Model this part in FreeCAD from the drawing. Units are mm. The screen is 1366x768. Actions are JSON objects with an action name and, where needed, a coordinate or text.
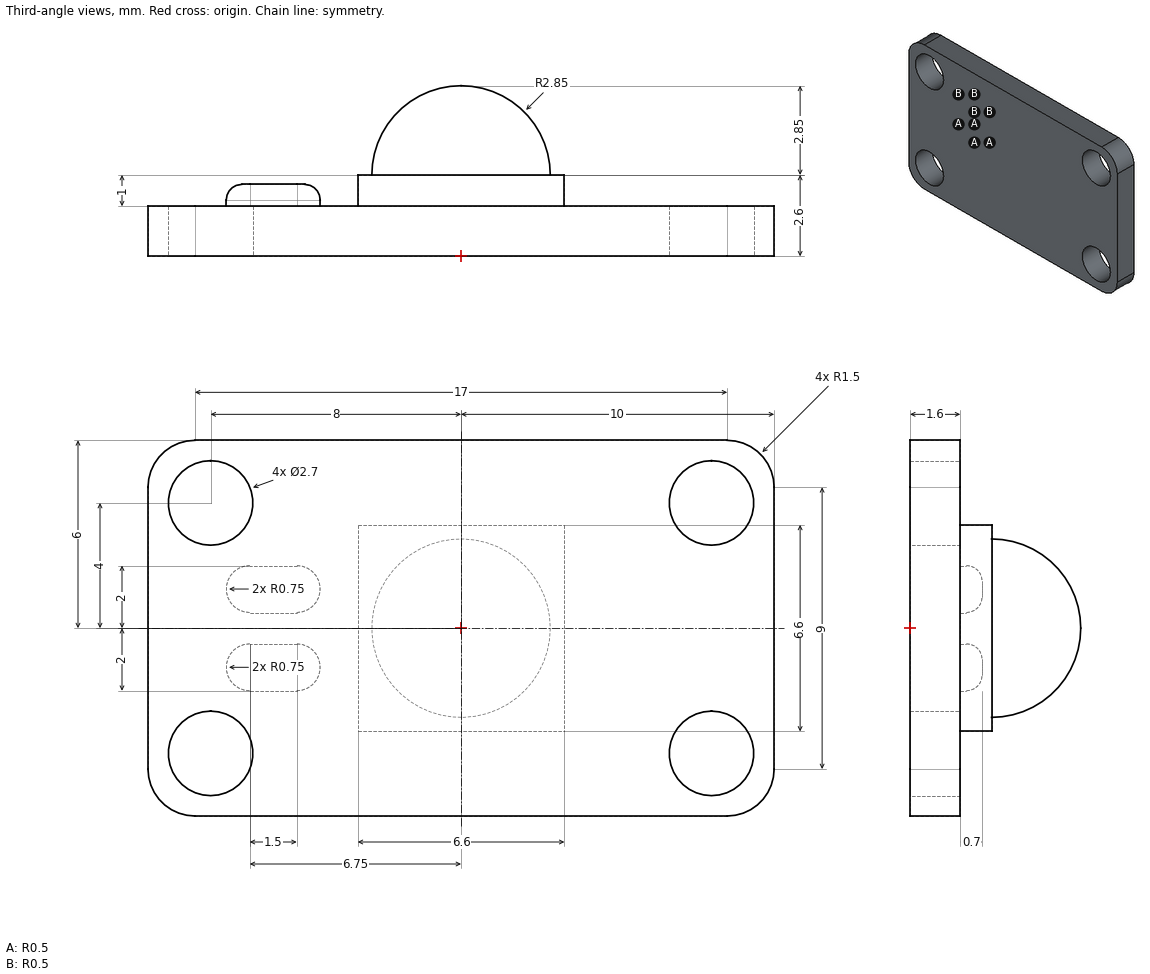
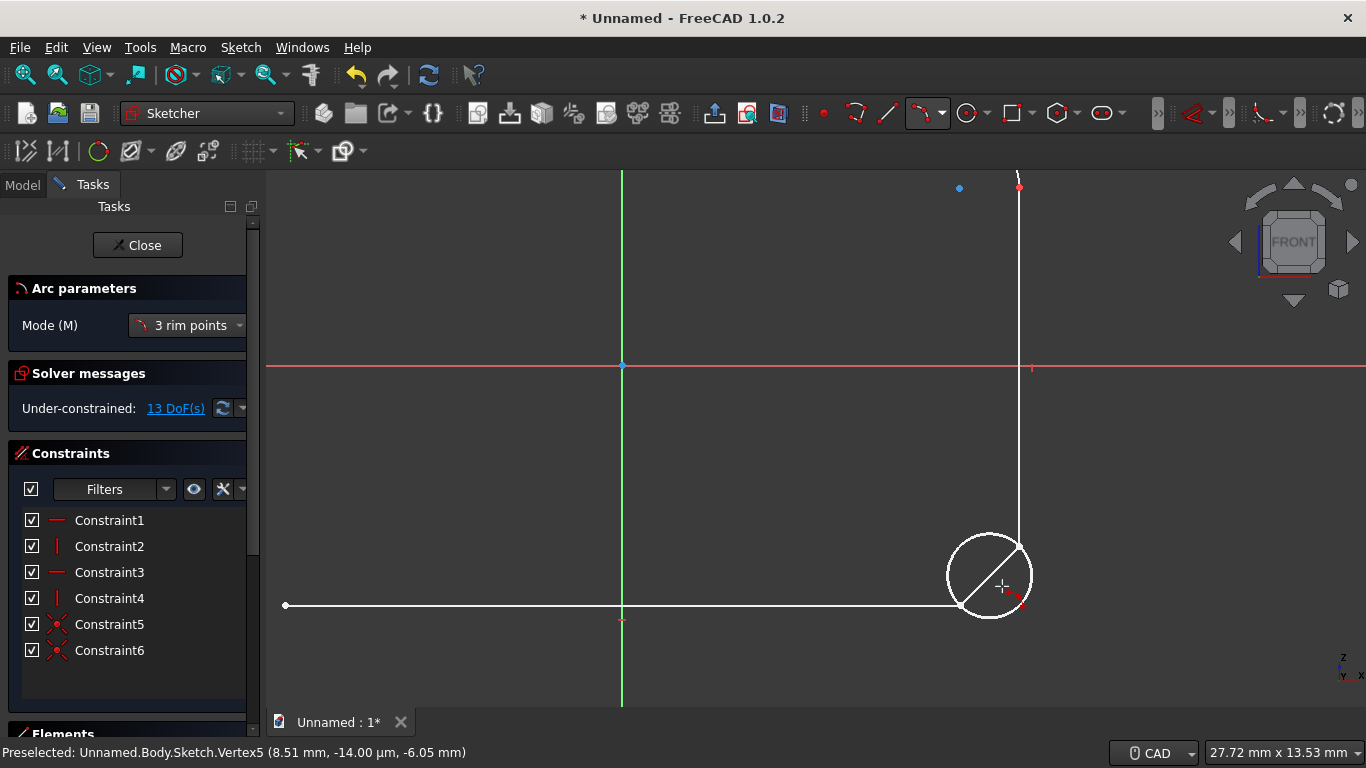
{"action": "left_click", "coordinate": [1002, 586]}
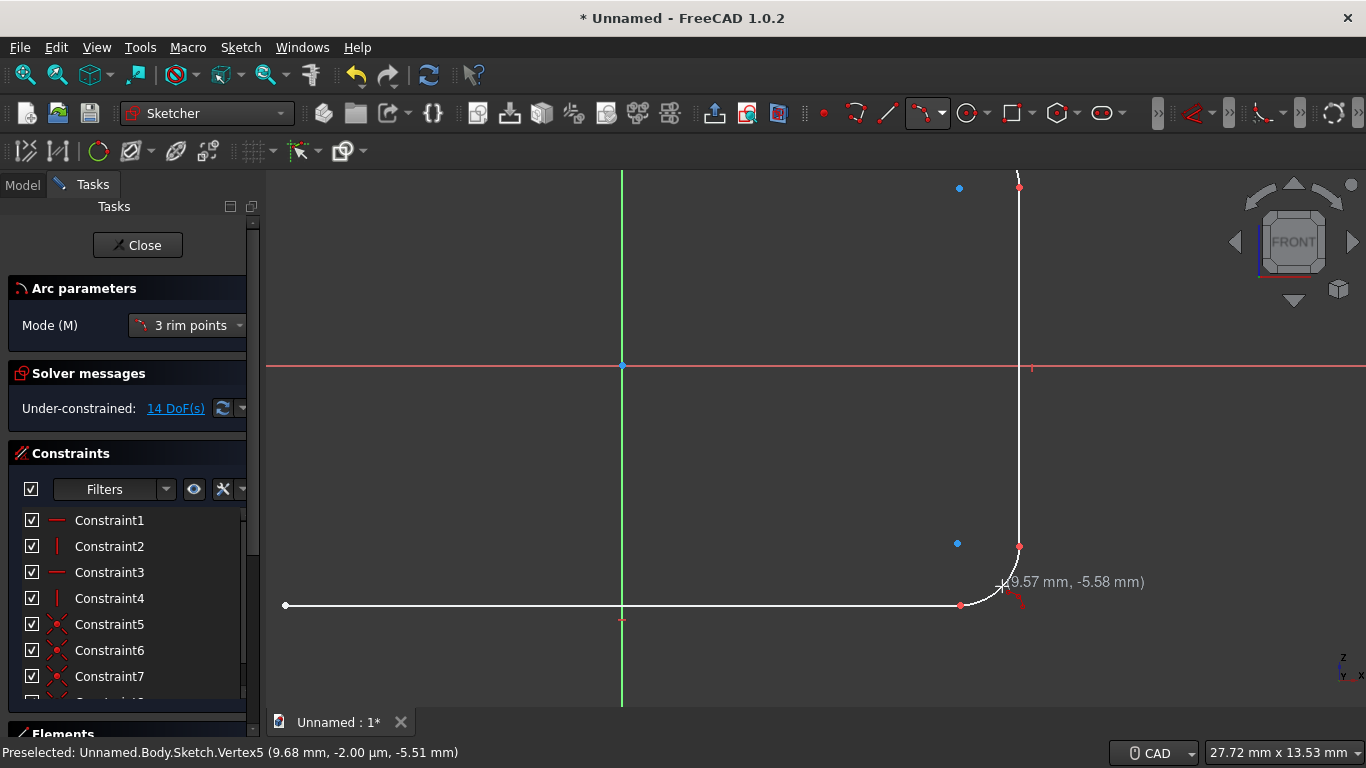
{"action": "scroll", "coordinate": [1002, 587], "scroll_direction": "down", "scroll_amount": 2}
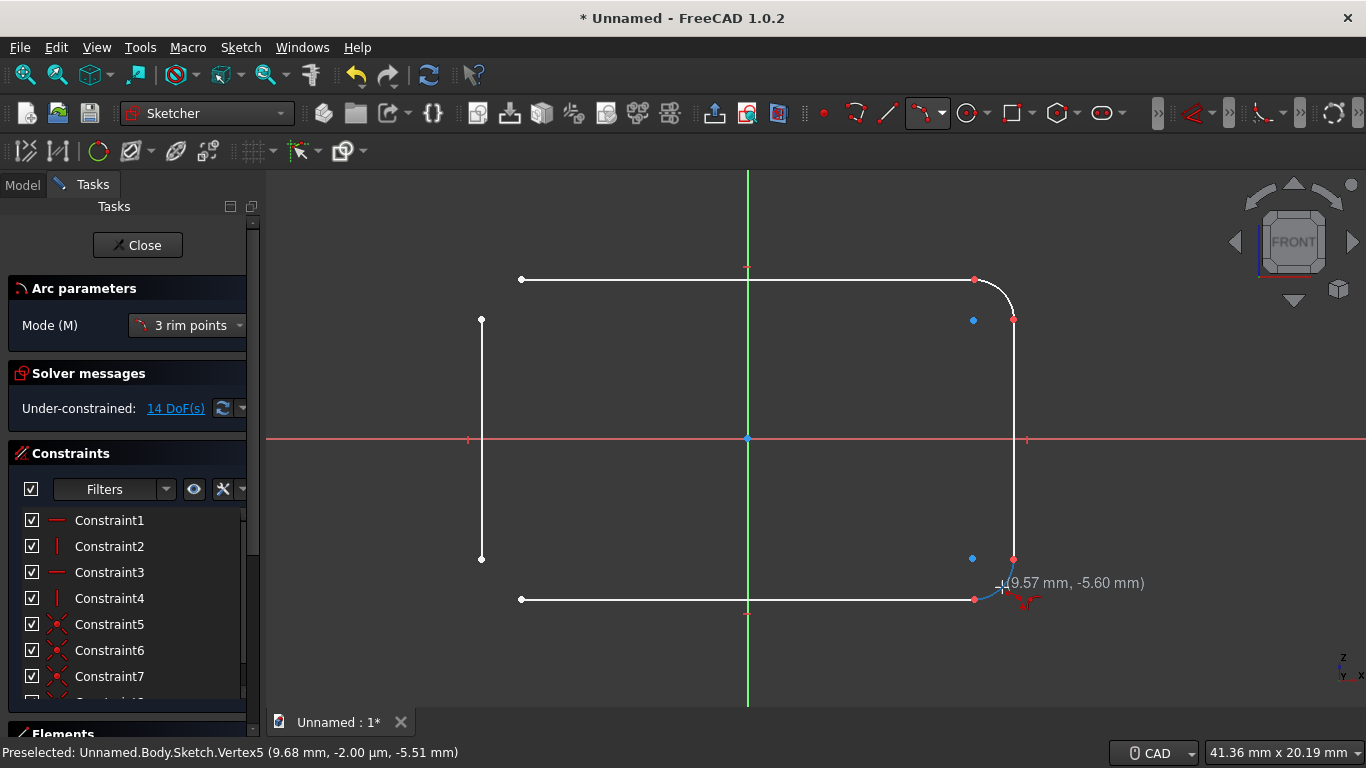
{"action": "left_click", "coordinate": [522, 600]}
{"action": "left_click", "coordinate": [482, 560]}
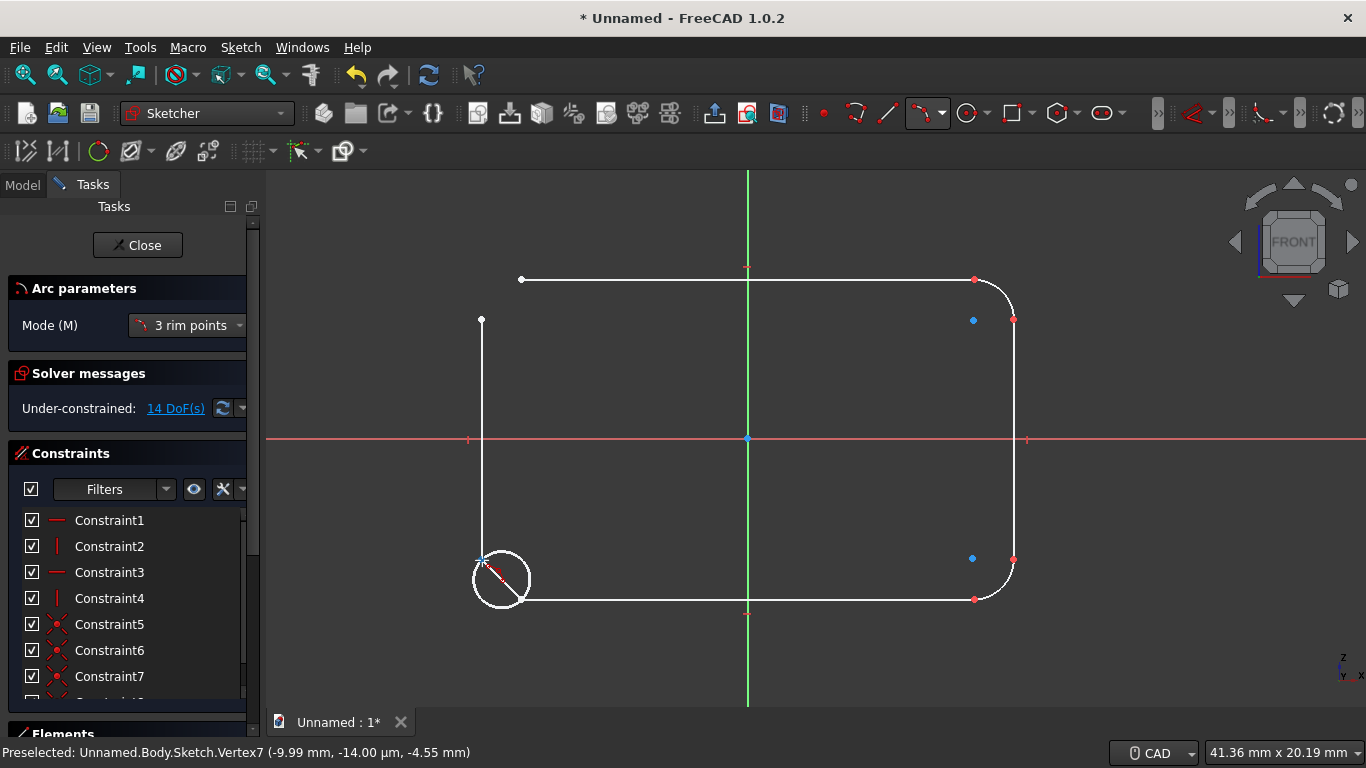
{"action": "scroll", "coordinate": [493, 587], "scroll_direction": "up", "scroll_amount": 2}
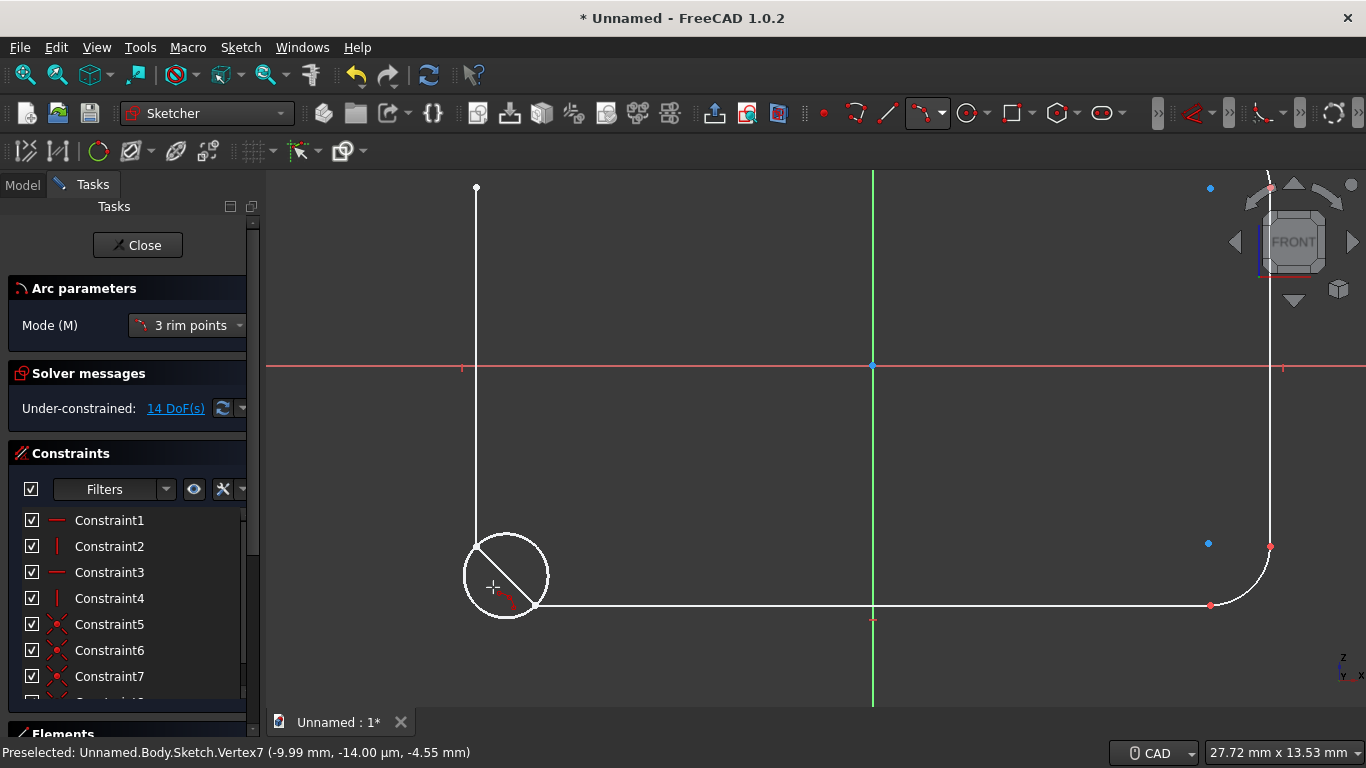
{"action": "left_click", "coordinate": [493, 586]}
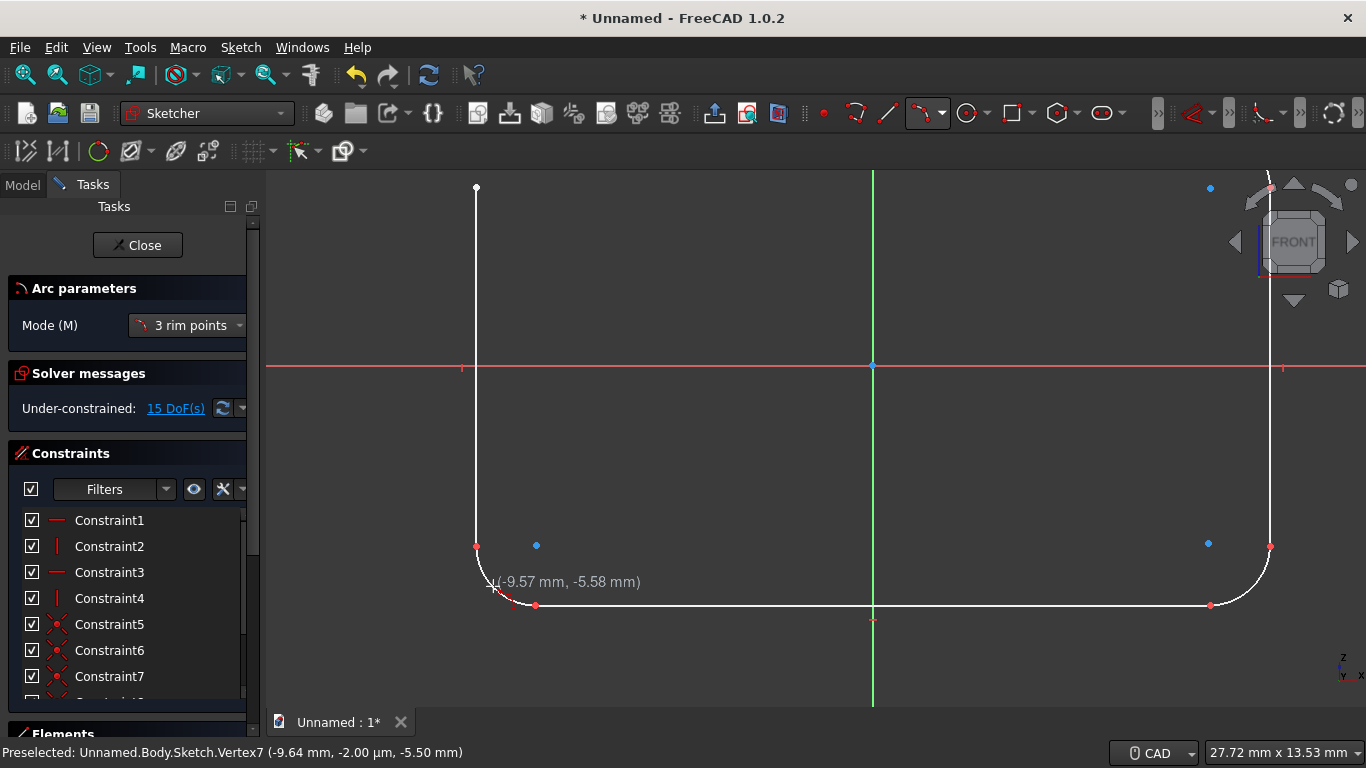
{"action": "scroll", "coordinate": [493, 587], "scroll_direction": "down", "scroll_amount": 2}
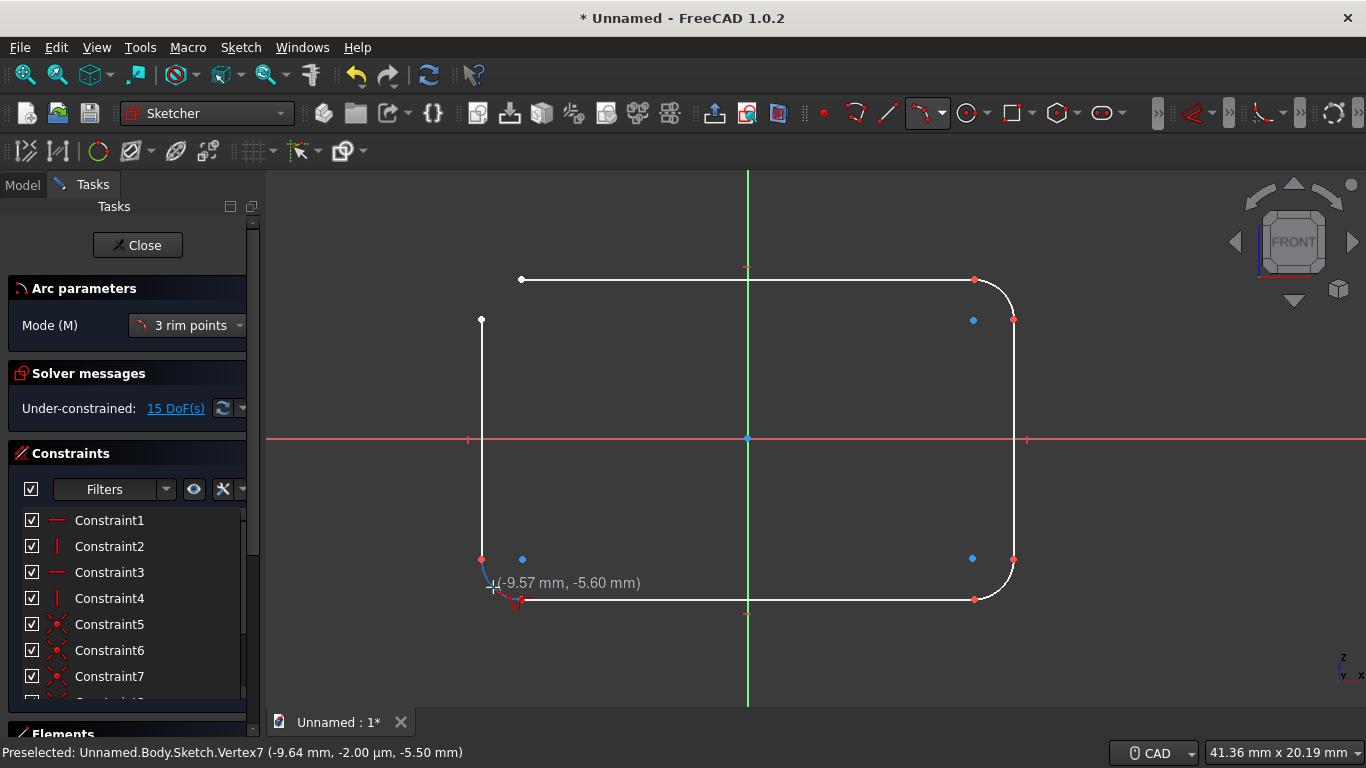
{"action": "left_click", "coordinate": [482, 320]}
{"action": "left_click", "coordinate": [522, 280]}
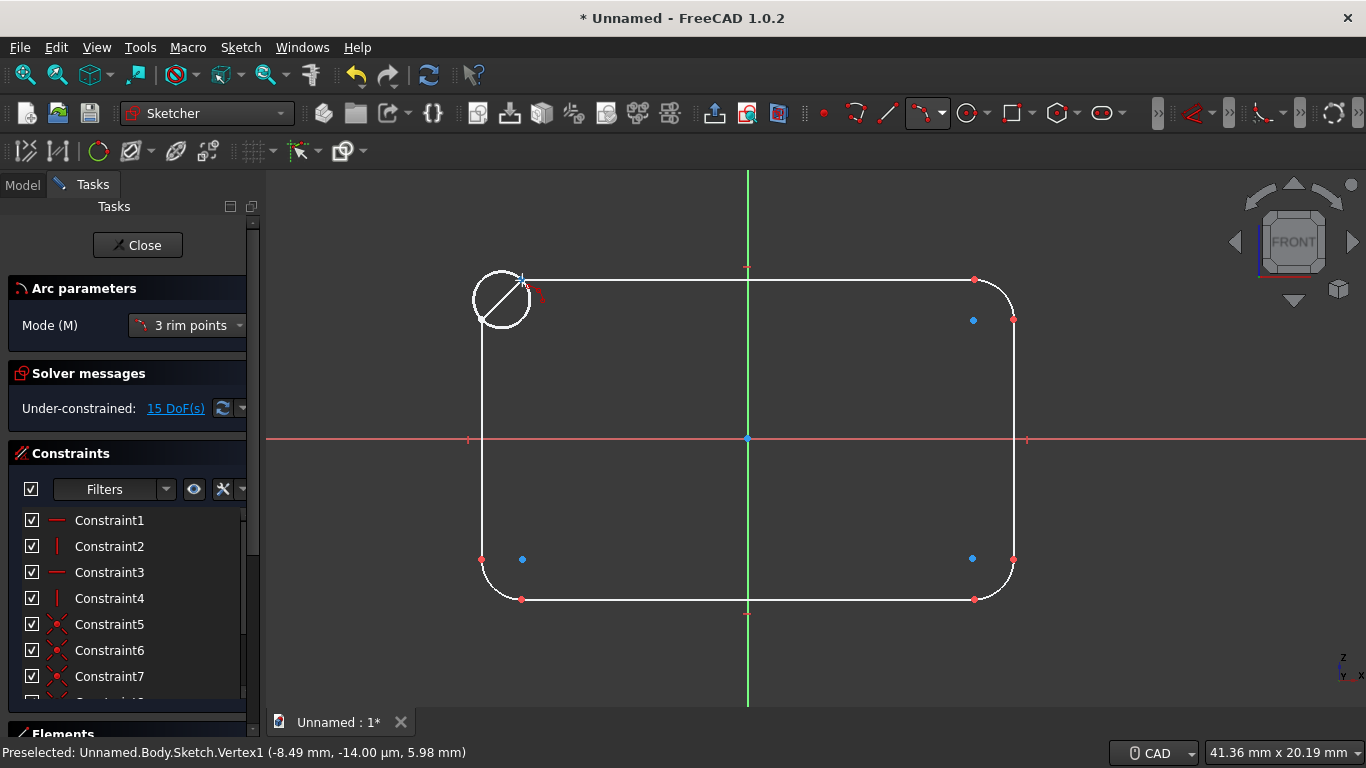
{"action": "scroll", "coordinate": [493, 291], "scroll_direction": "up", "scroll_amount": 2}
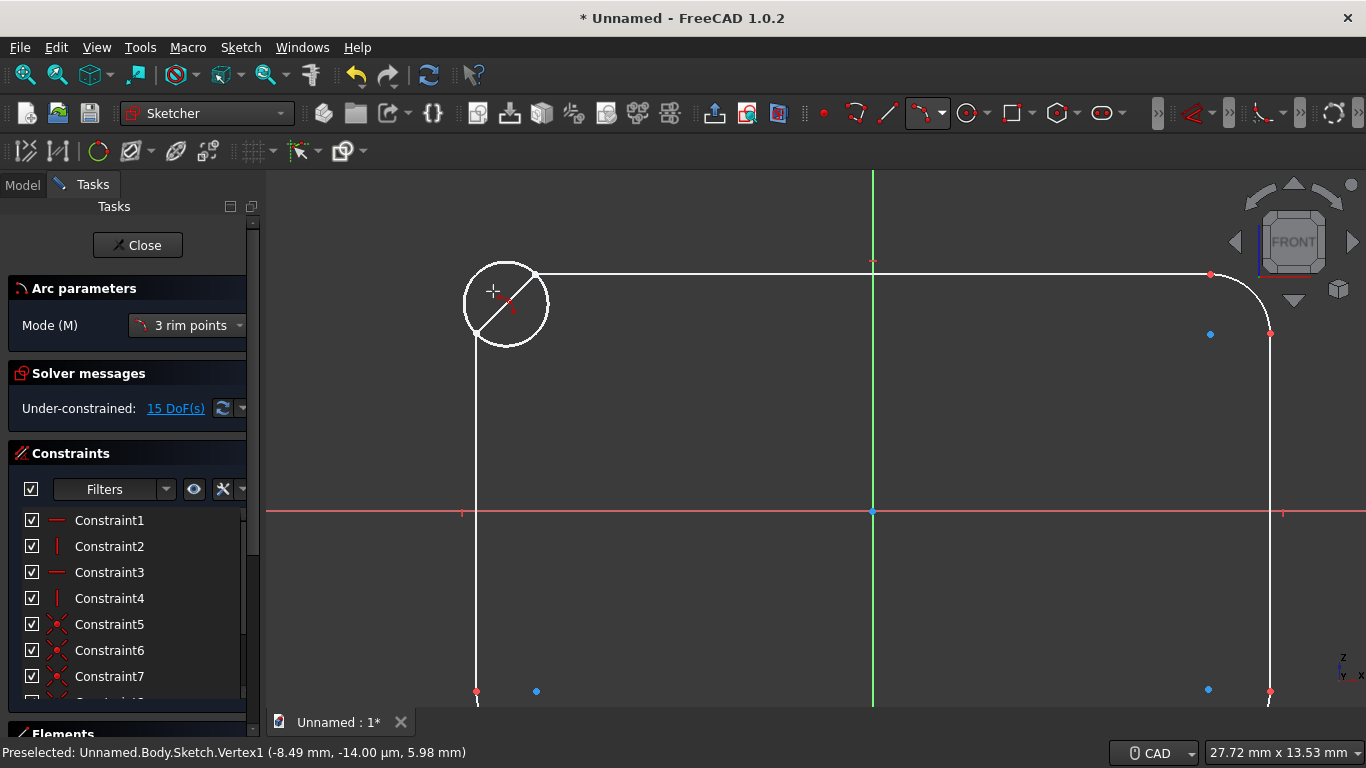
{"action": "left_click", "coordinate": [493, 291]}
{"action": "key", "text": "Escape"}